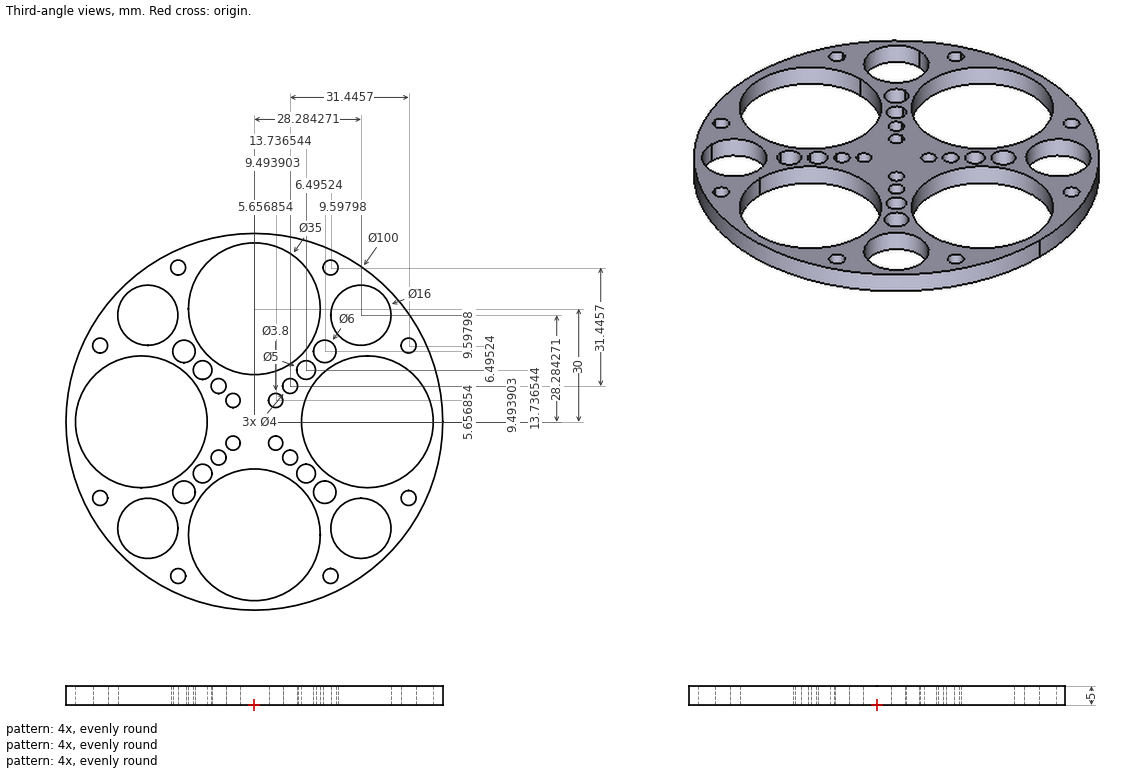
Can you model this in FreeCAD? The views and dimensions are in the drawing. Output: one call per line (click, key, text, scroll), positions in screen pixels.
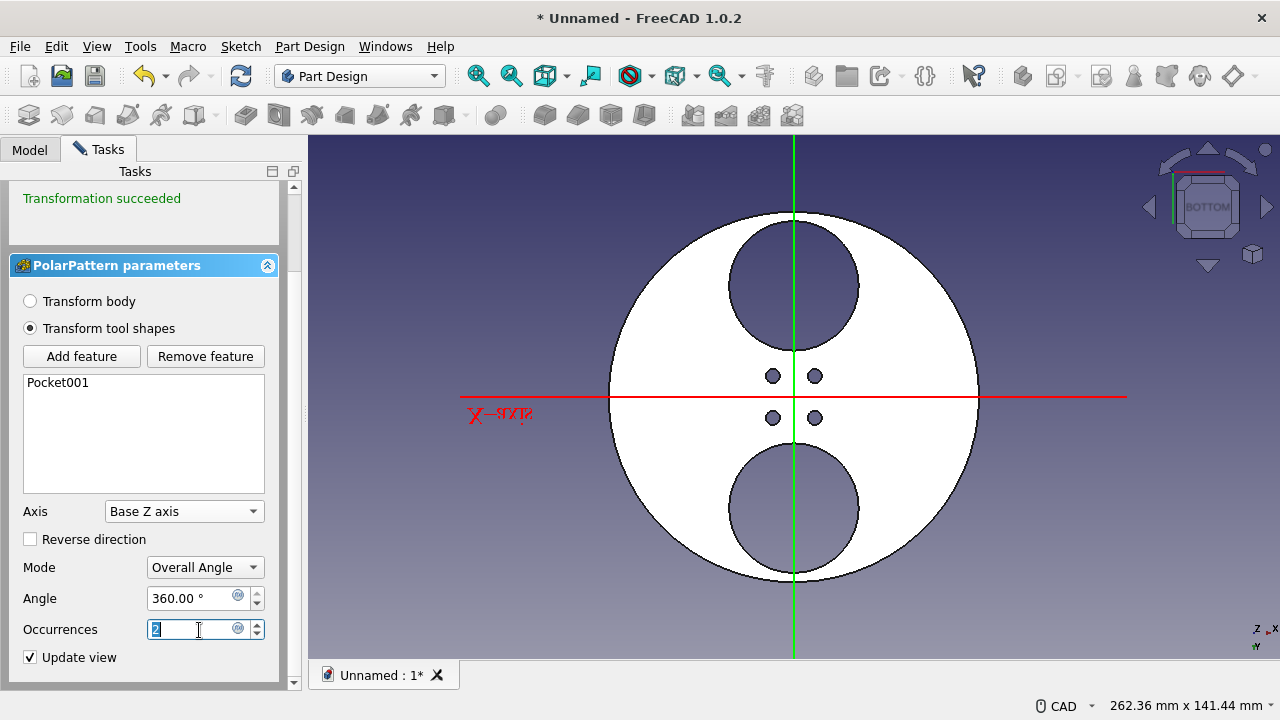
text(4)
key(Tab)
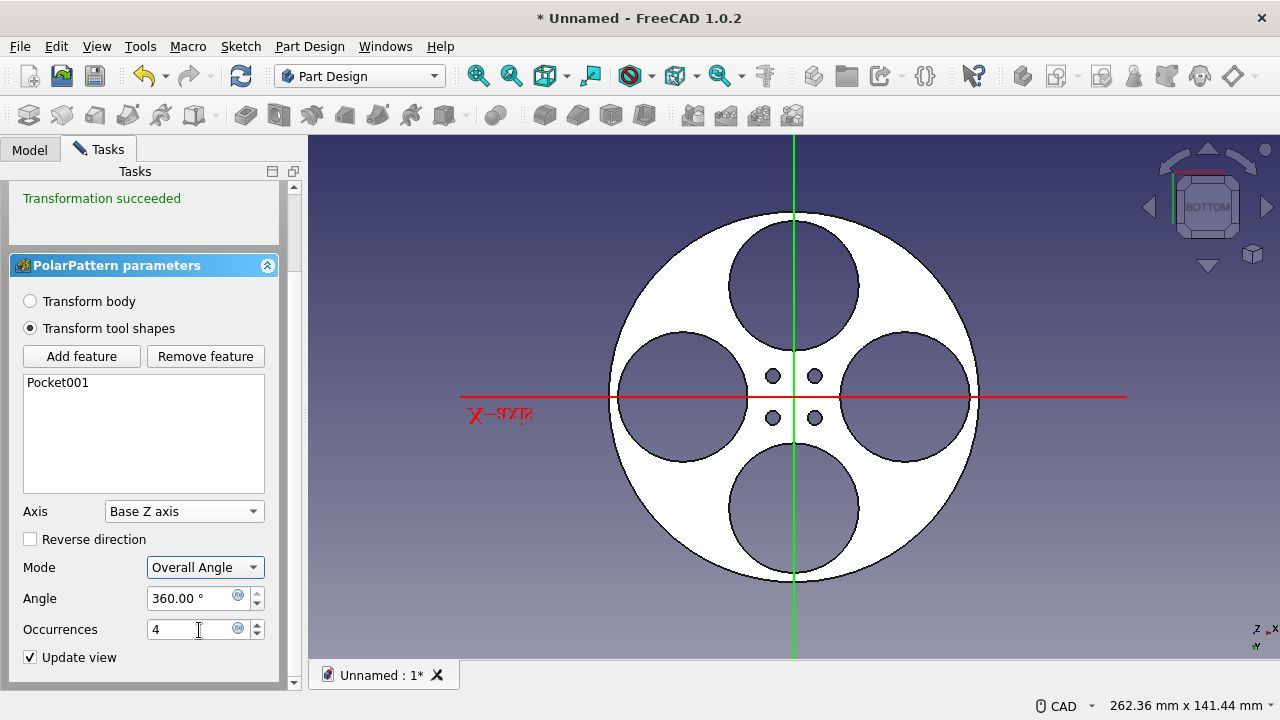
scroll(294, 436, up, 3)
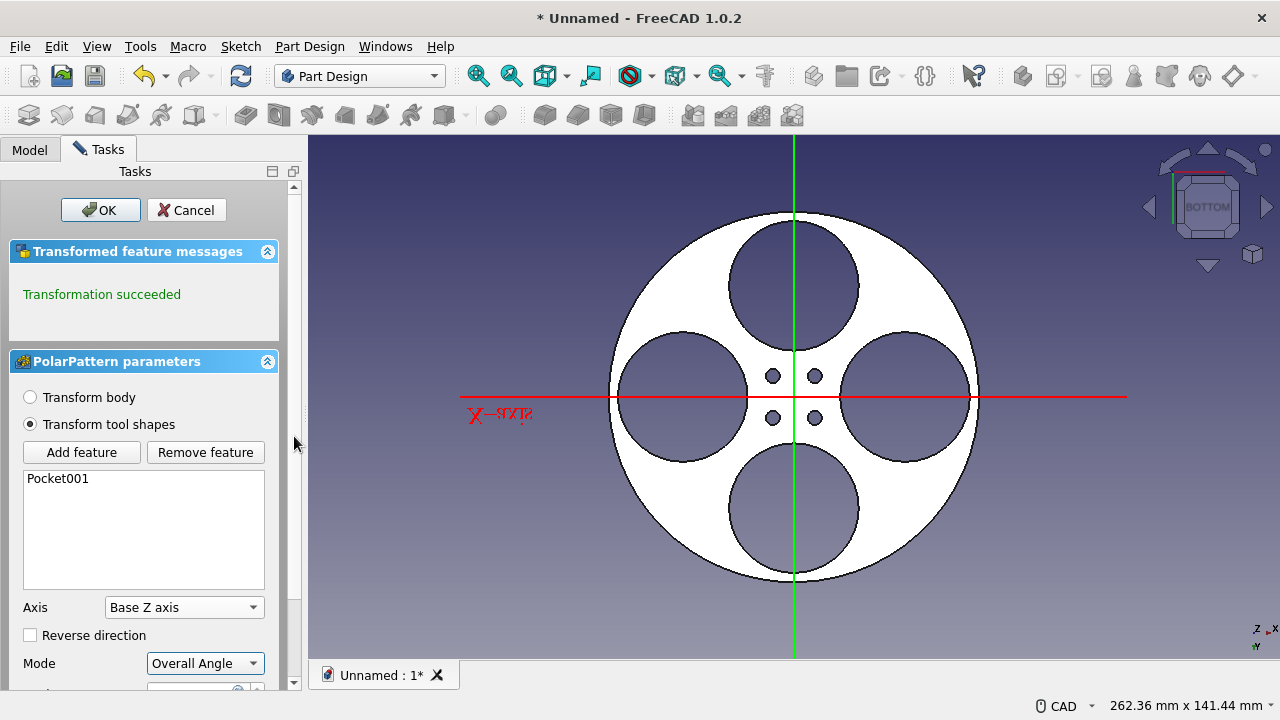
click(101, 210)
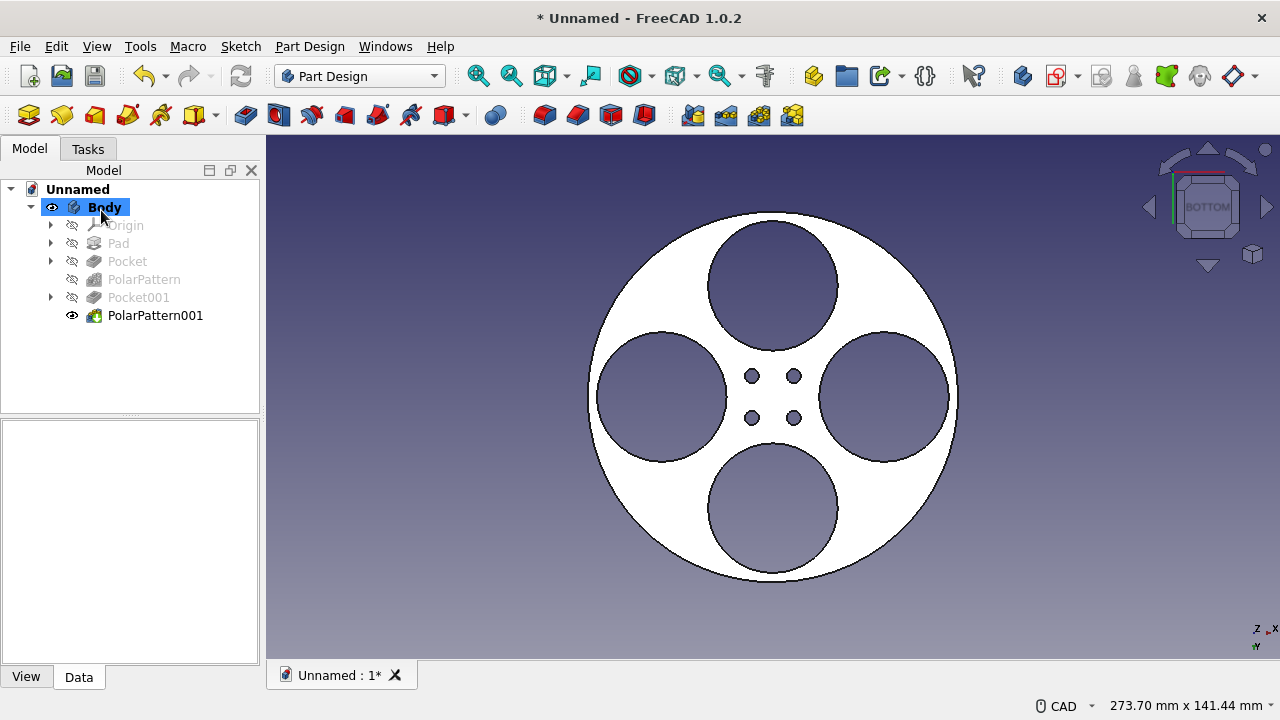
click(1056, 76)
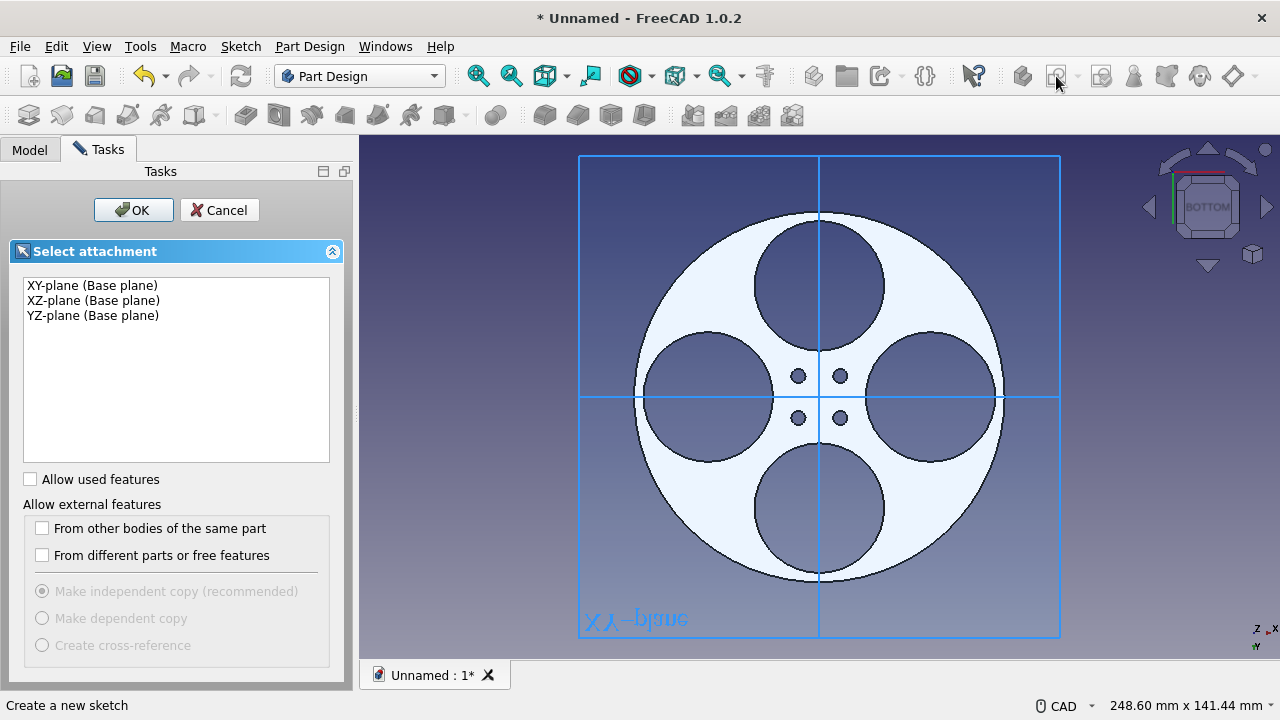
click(84, 286)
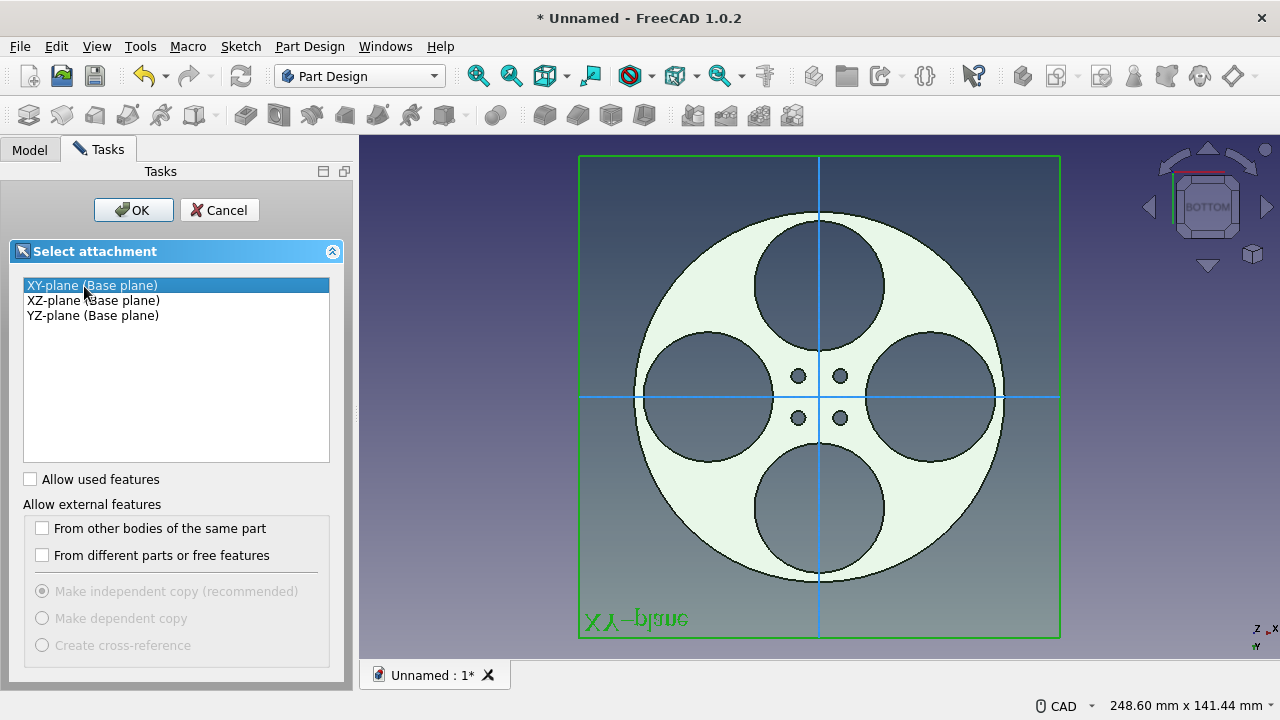
click(134, 210)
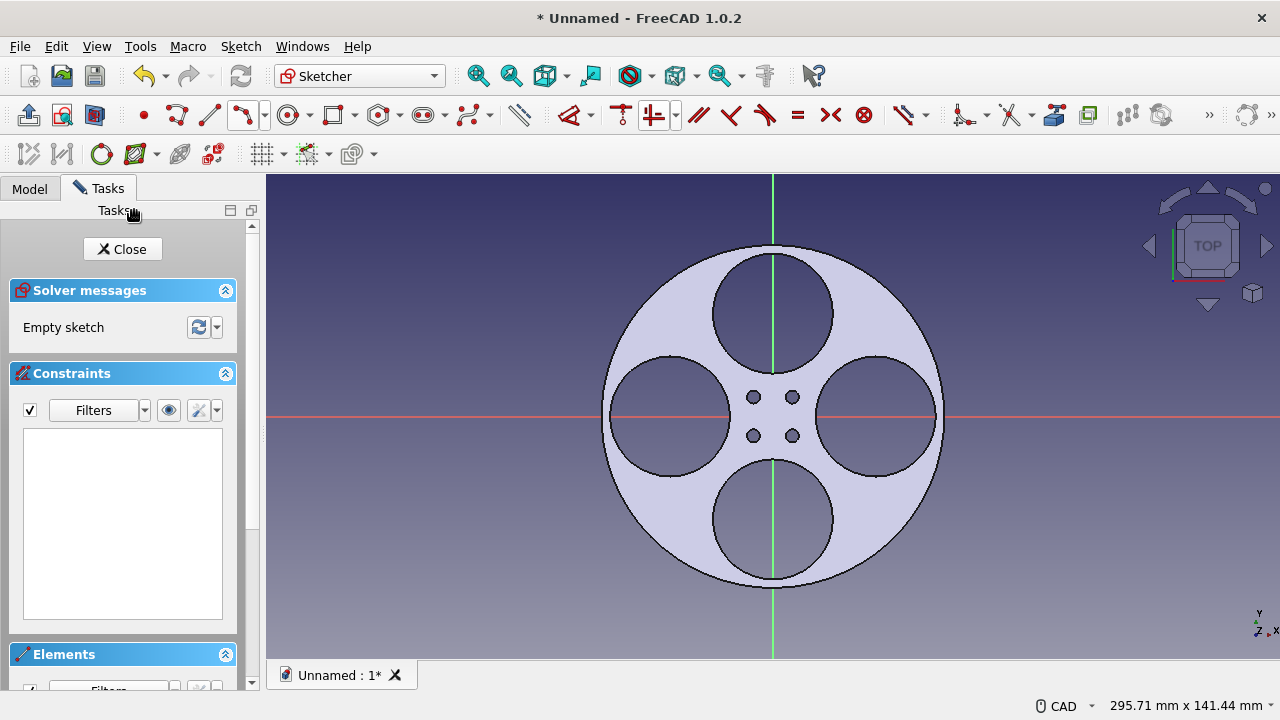
click(95, 116)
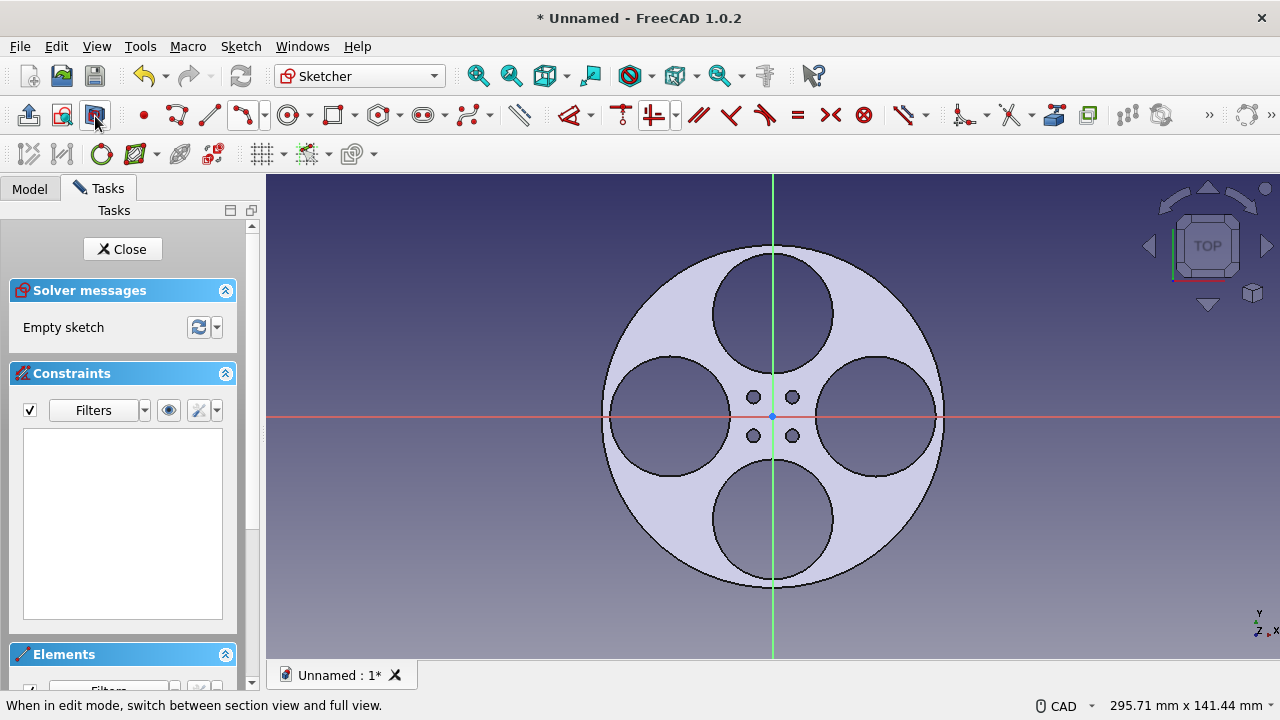
scroll(962, 283, up, 4)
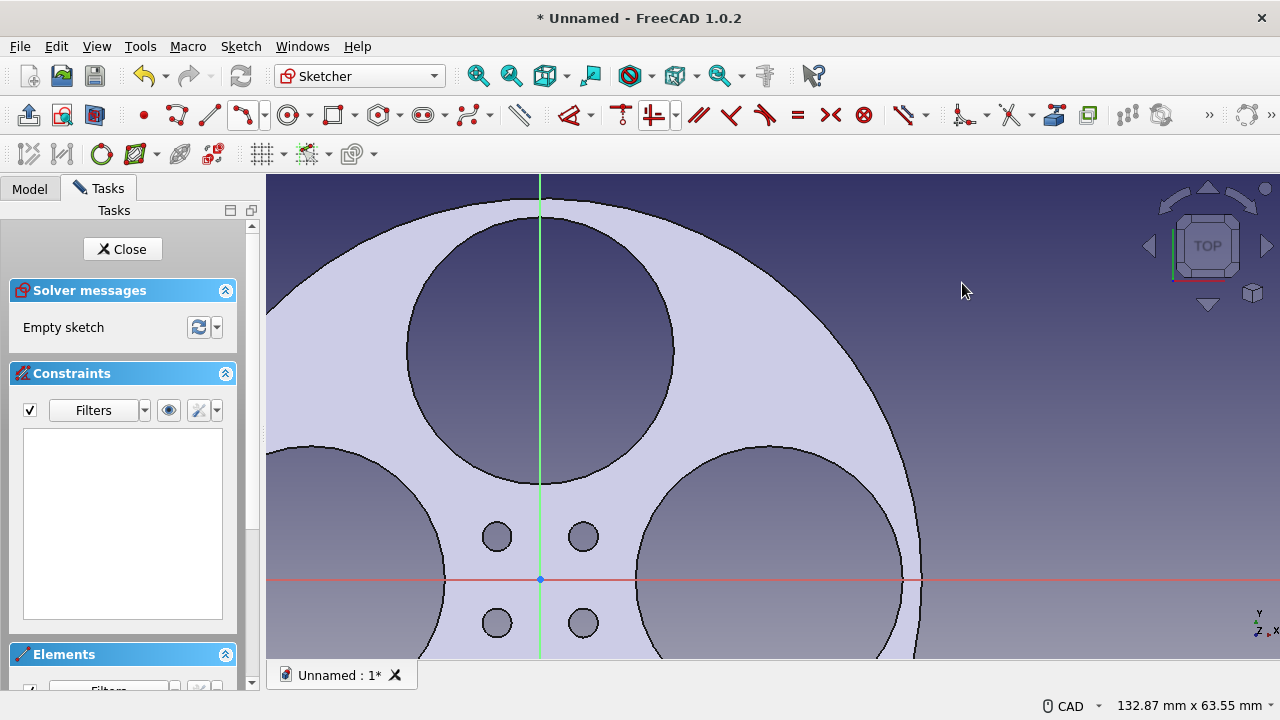
click(288, 116)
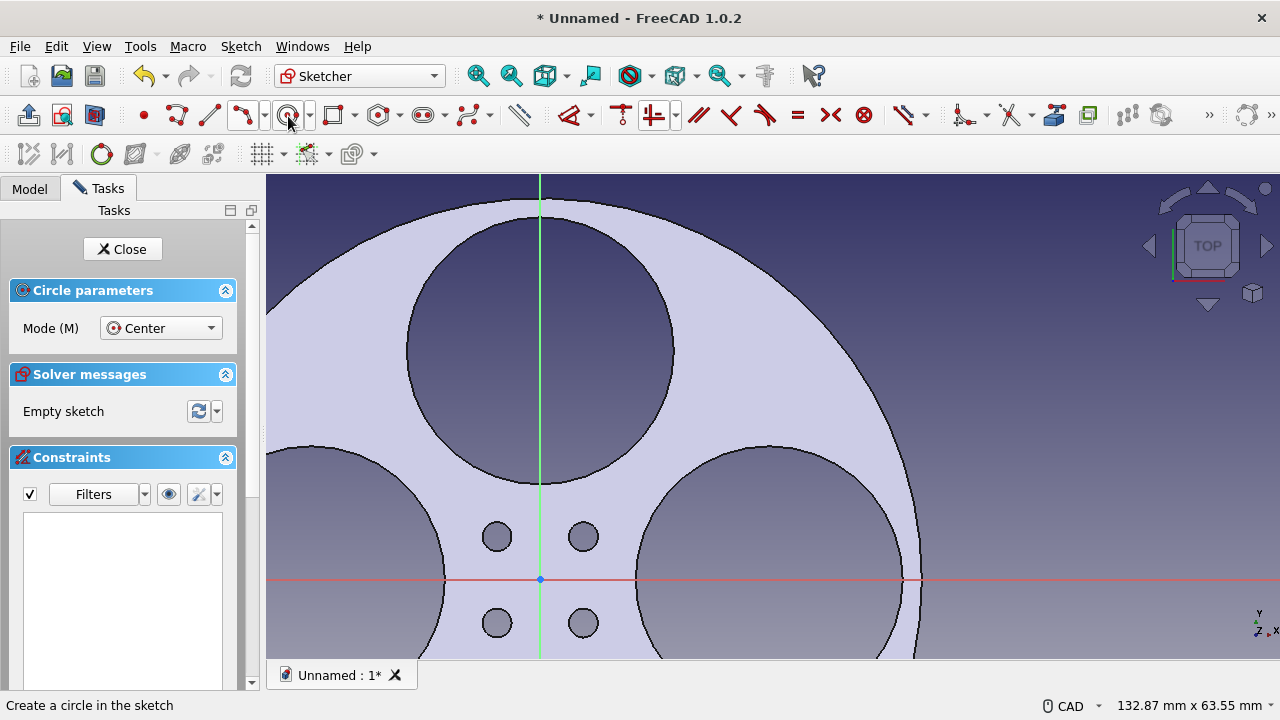
click(756, 364)
click(799, 321)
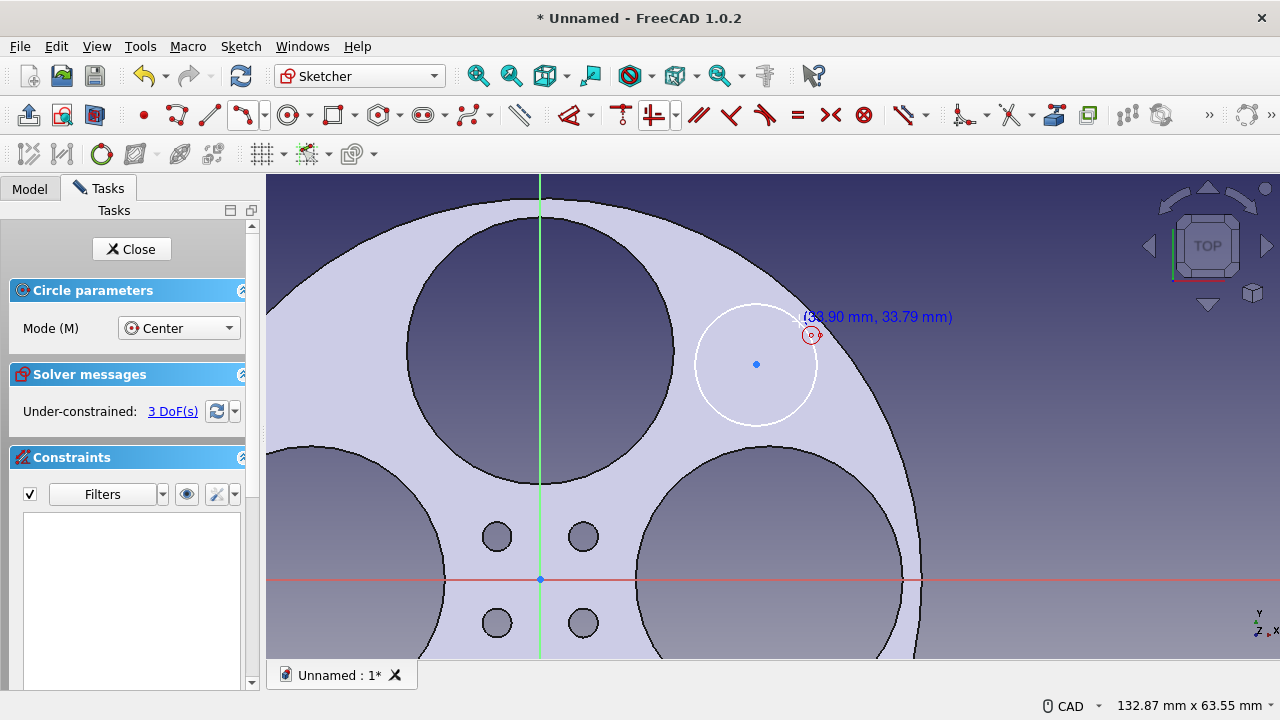
click(683, 437)
click(699, 421)